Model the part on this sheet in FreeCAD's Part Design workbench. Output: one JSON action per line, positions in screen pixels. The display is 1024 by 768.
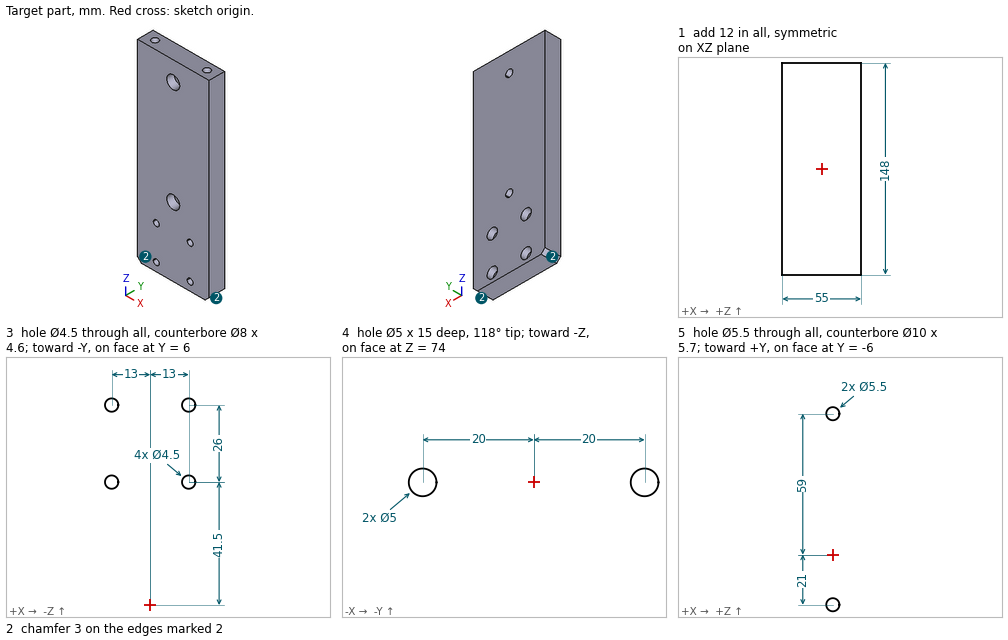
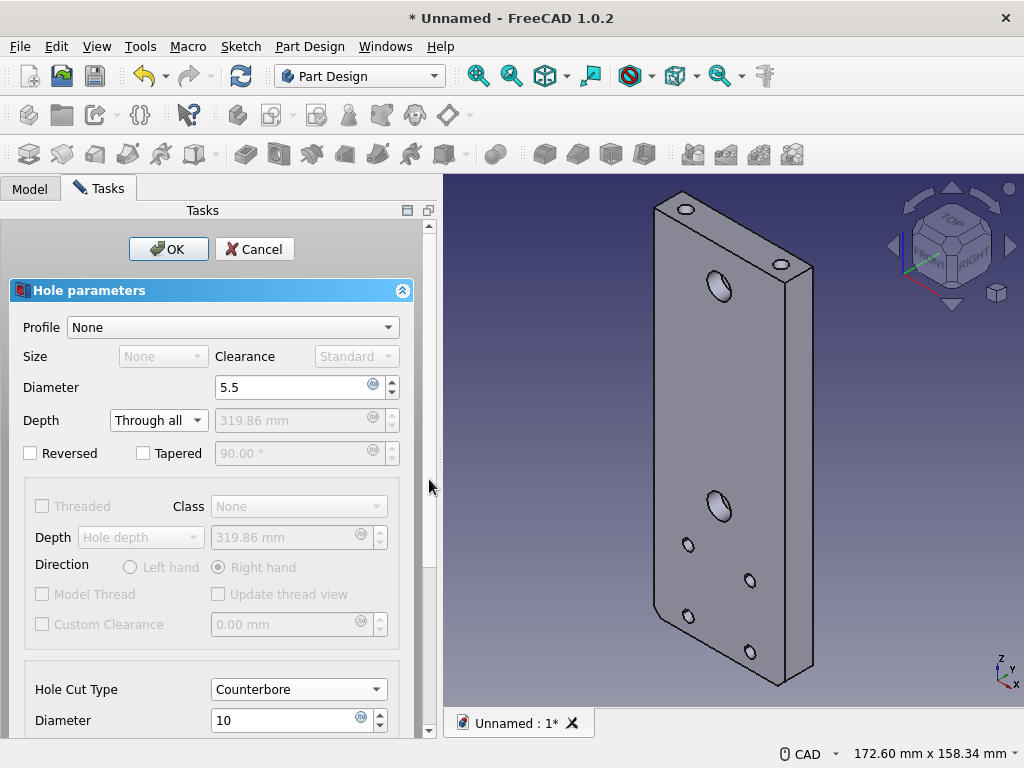
{"action": "left_click", "coordinate": [169, 249]}